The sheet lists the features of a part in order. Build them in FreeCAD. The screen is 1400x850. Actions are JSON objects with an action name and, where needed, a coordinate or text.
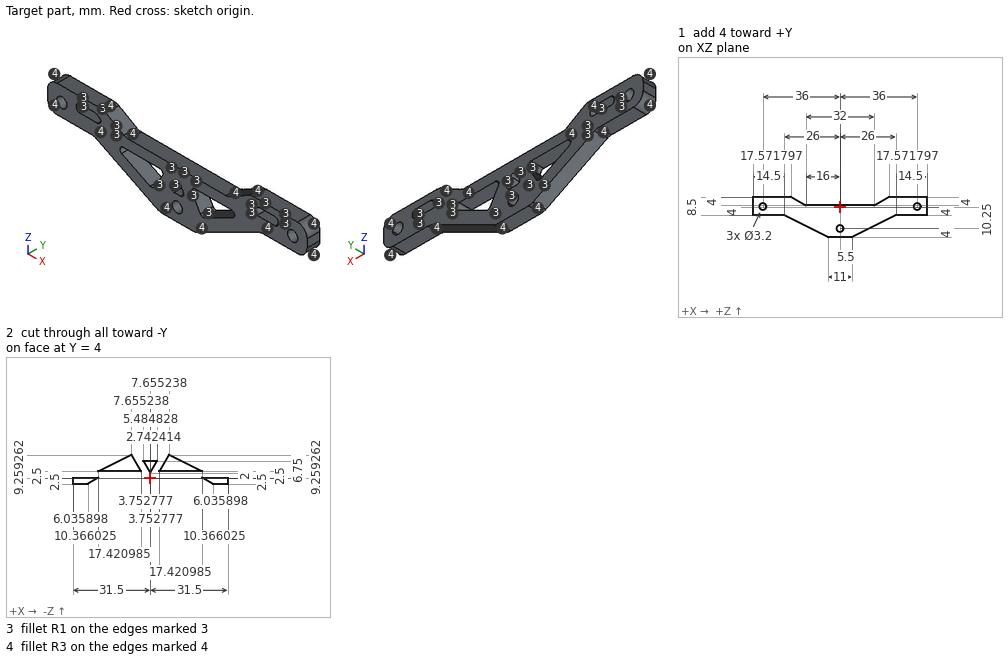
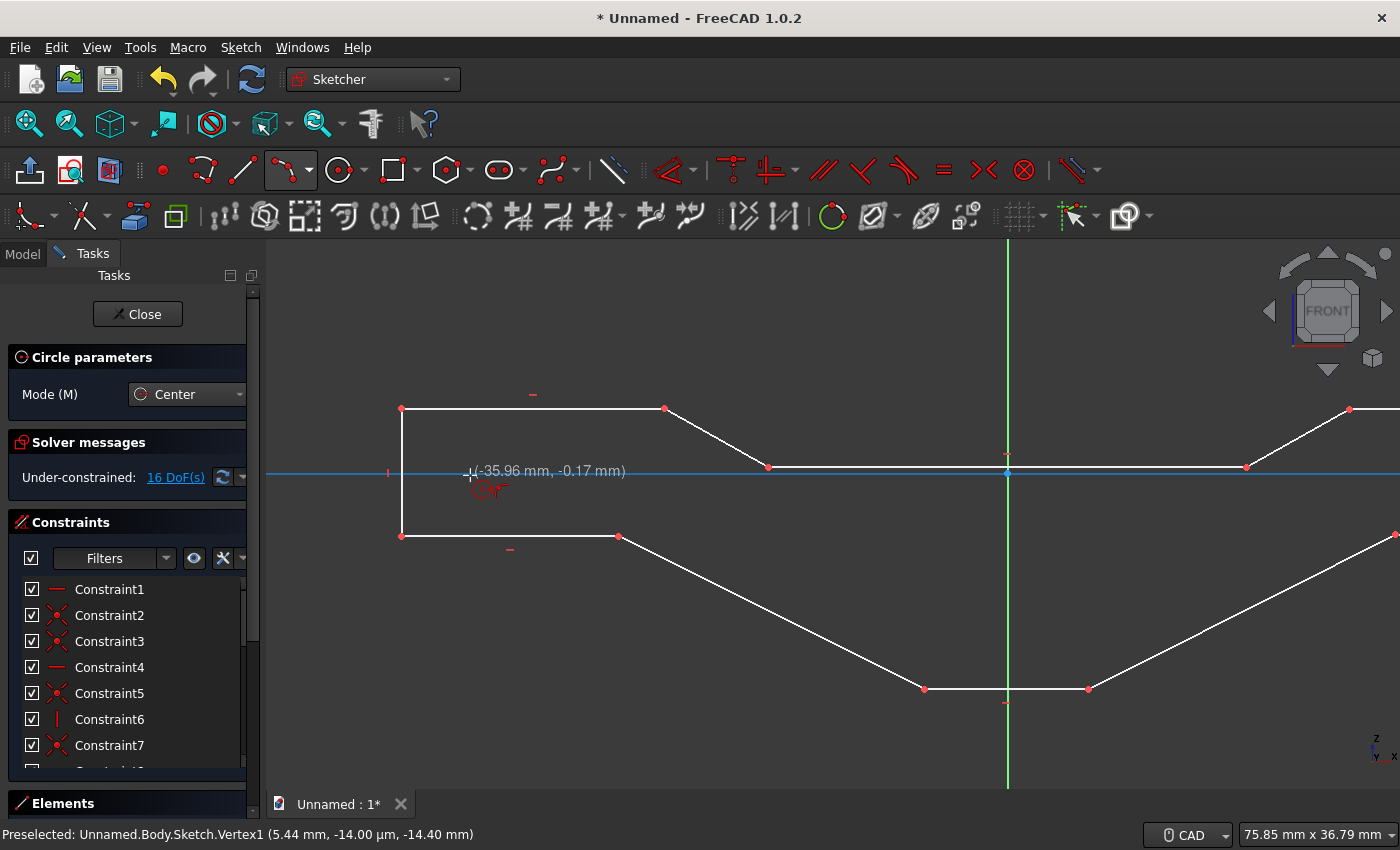
{"action": "left_click", "coordinate": [469, 474]}
{"action": "left_click", "coordinate": [486, 457]}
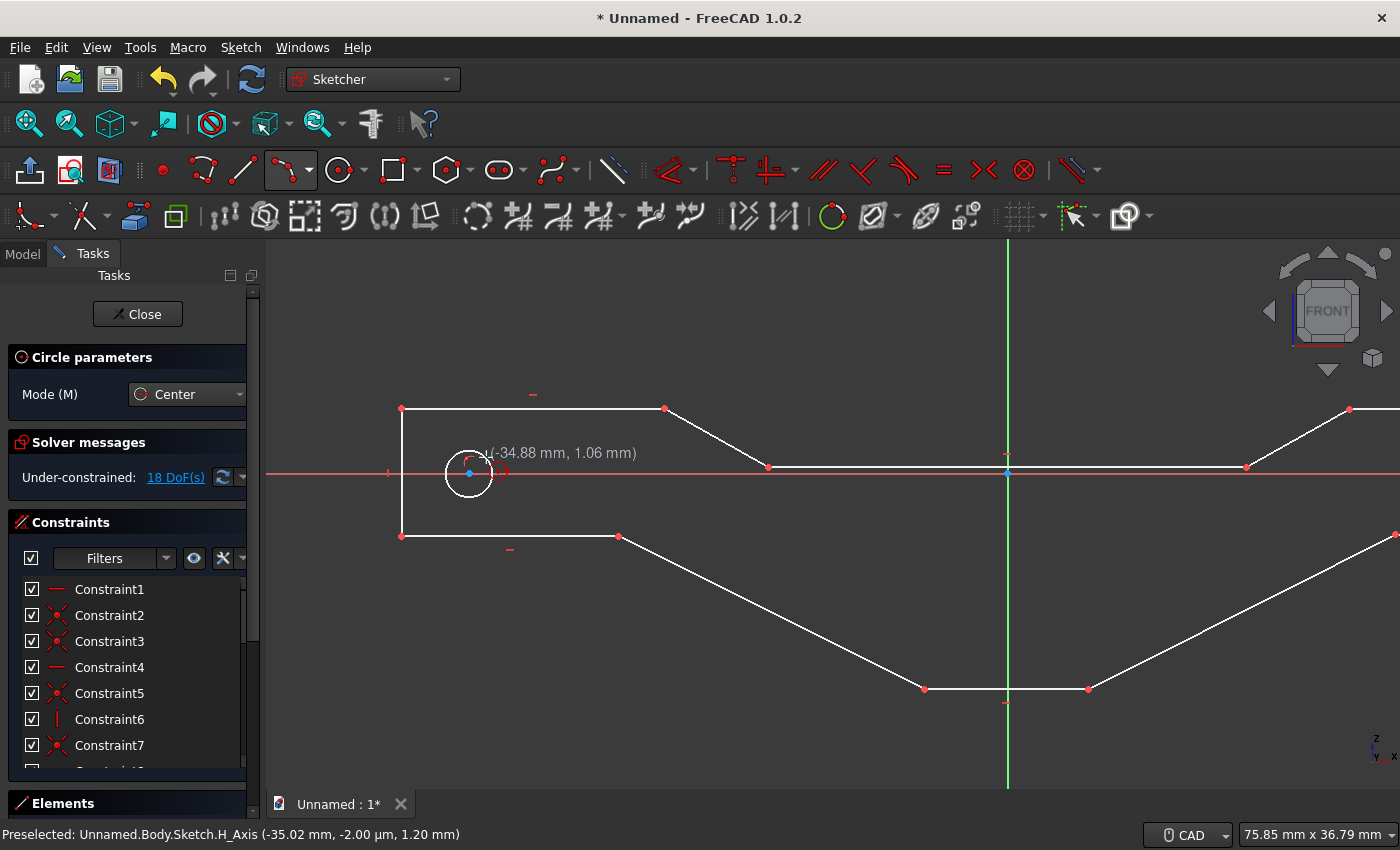
{"action": "scroll", "coordinate": [469, 474], "scroll_direction": "down", "scroll_amount": 3}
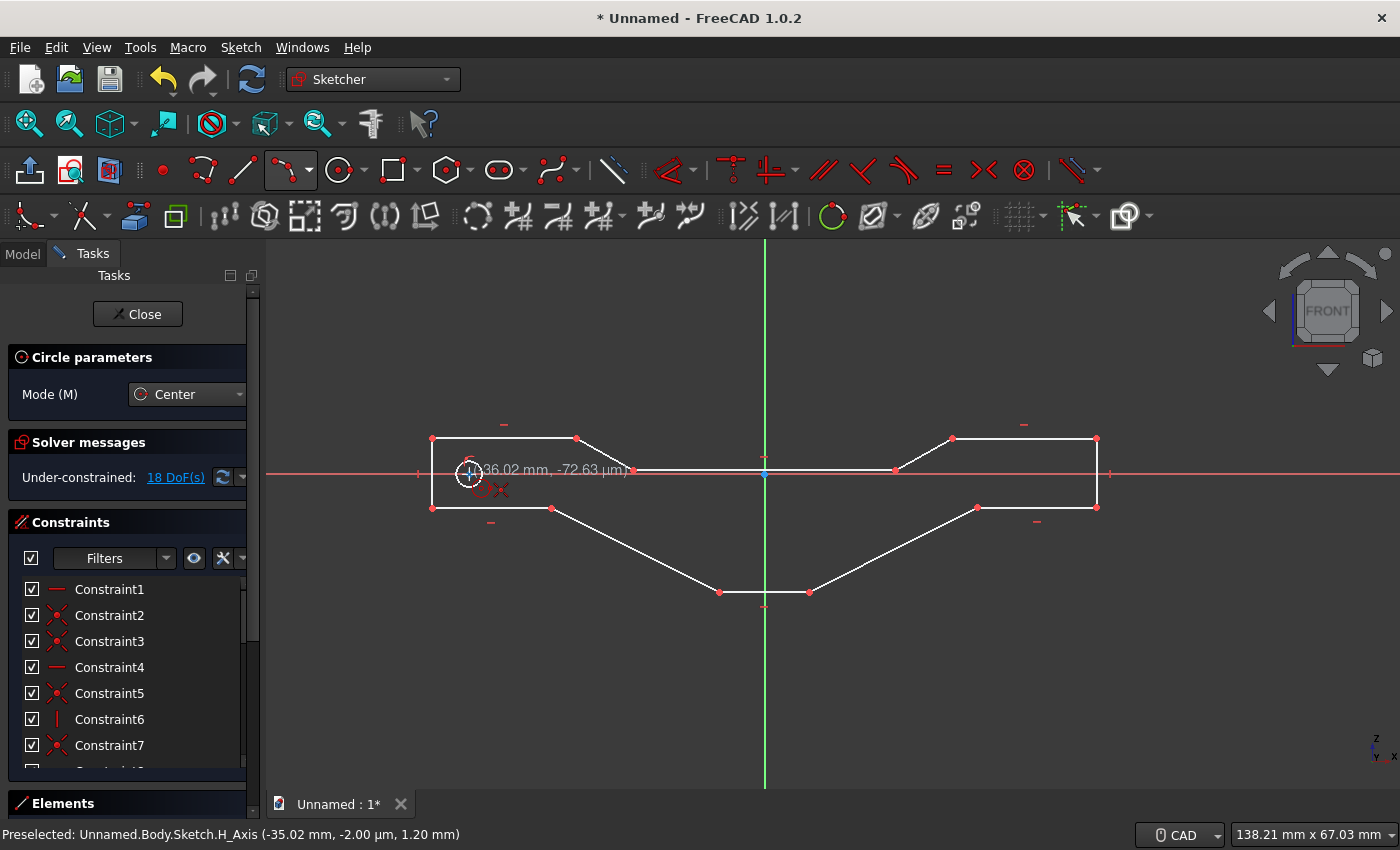
{"action": "scroll", "coordinate": [1060, 474], "scroll_direction": "up", "scroll_amount": 3}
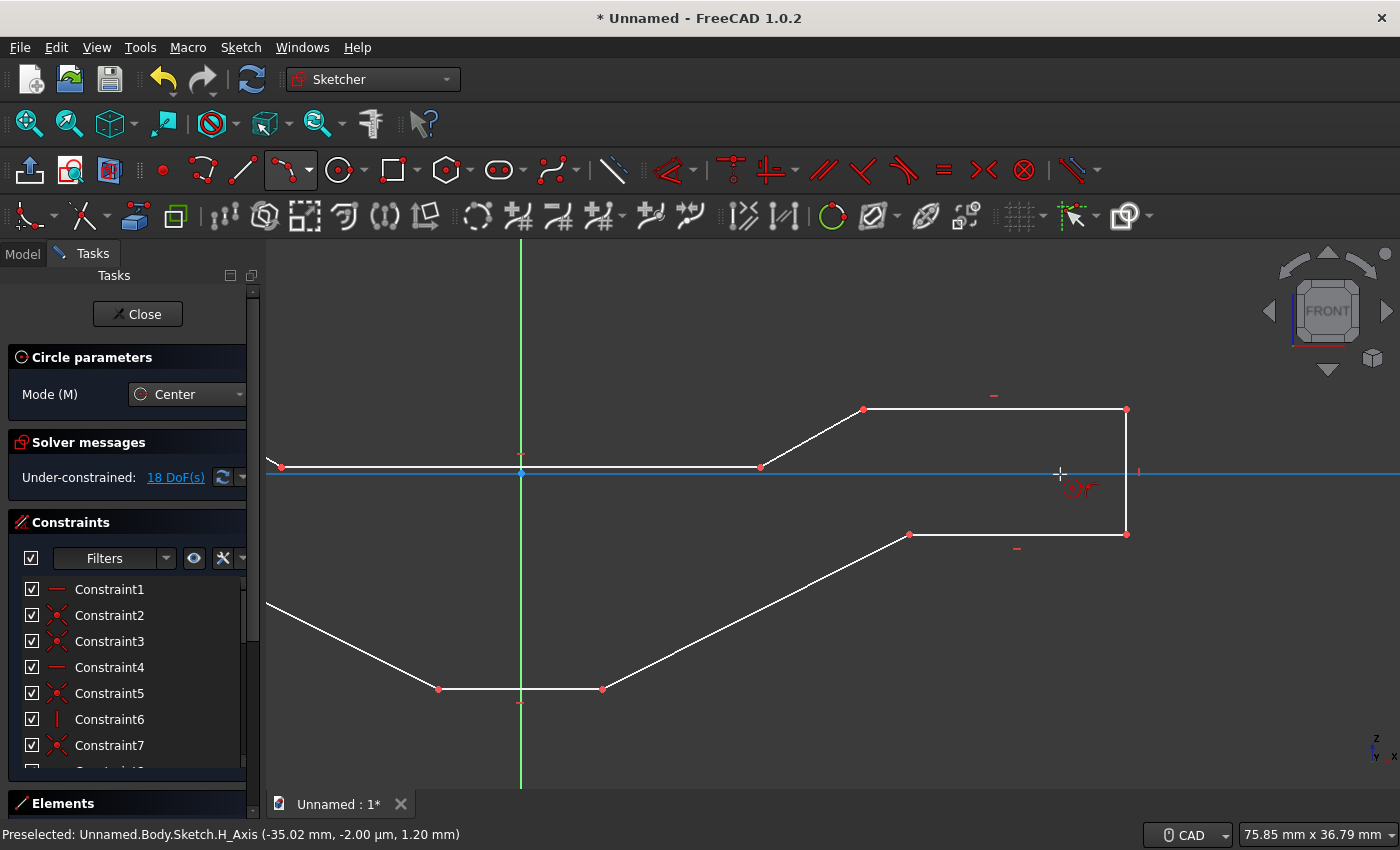
{"action": "left_click", "coordinate": [1059, 474]}
{"action": "left_click", "coordinate": [1076, 457]}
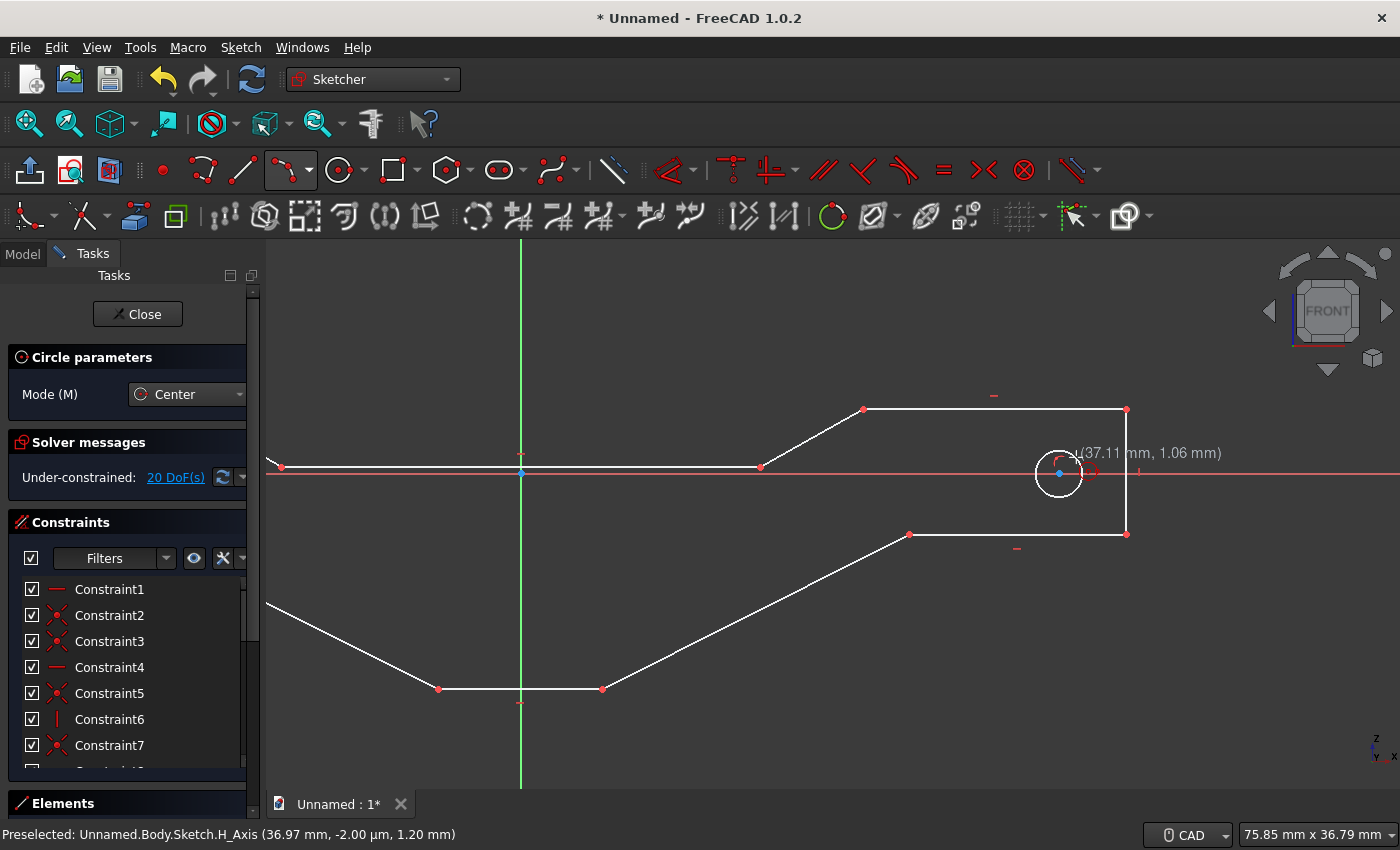
{"action": "left_click", "coordinate": [521, 627]}
{"action": "left_click", "coordinate": [538, 610]}
{"action": "key", "text": "Escape"}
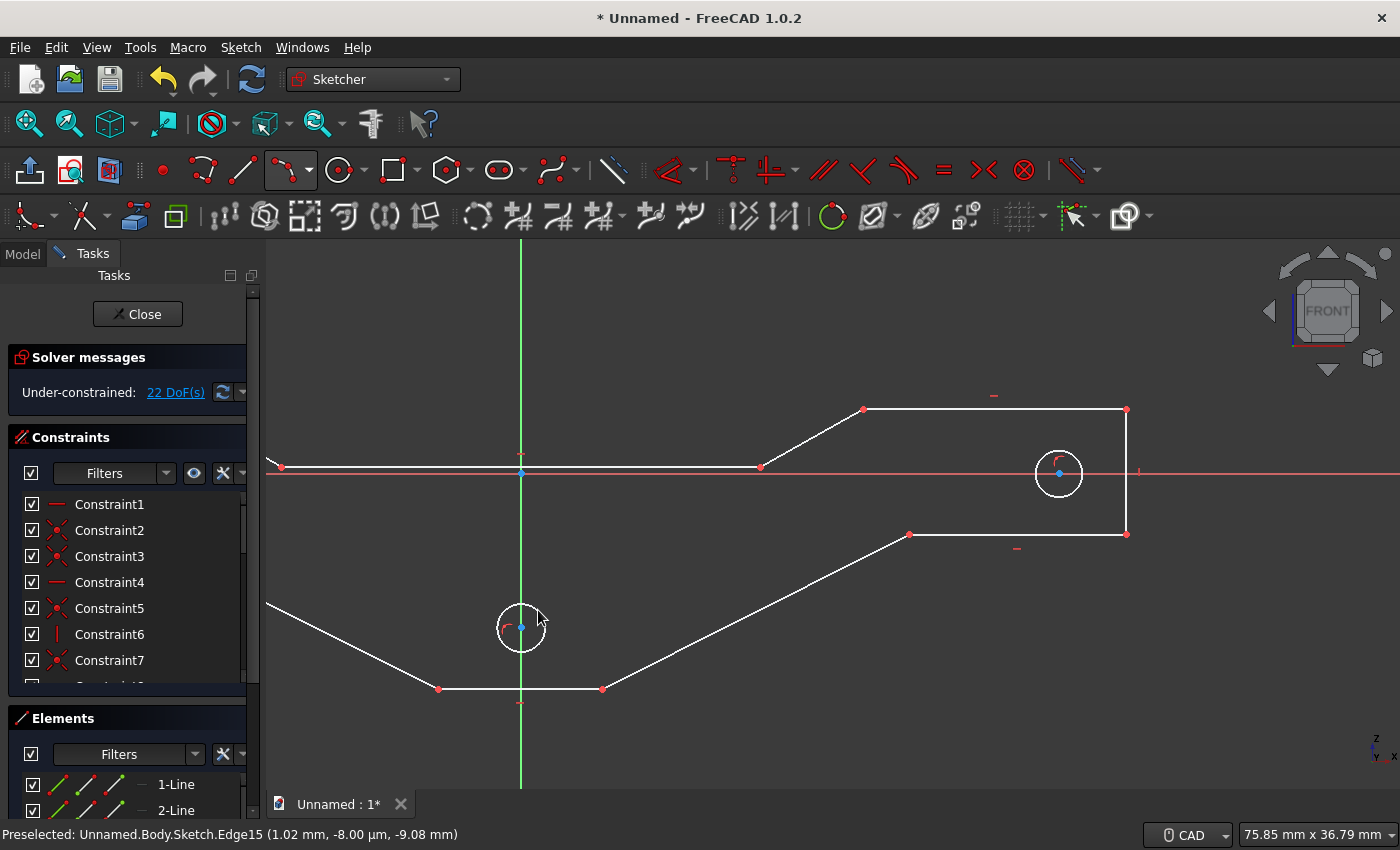
{"action": "scroll", "coordinate": [1060, 474], "scroll_direction": "down", "scroll_amount": 3}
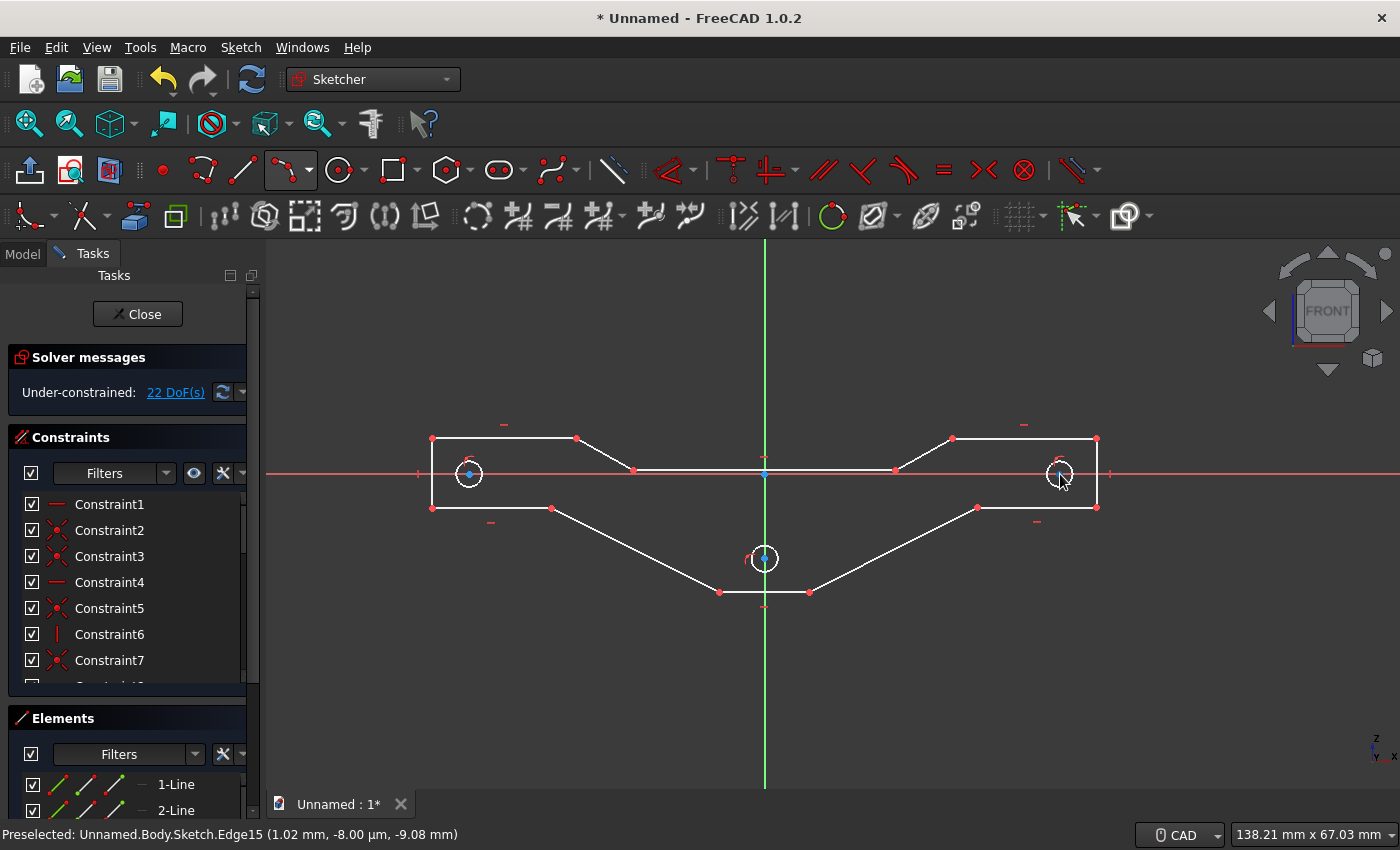
{"action": "scroll", "coordinate": [478, 465], "scroll_direction": "up", "scroll_amount": 3}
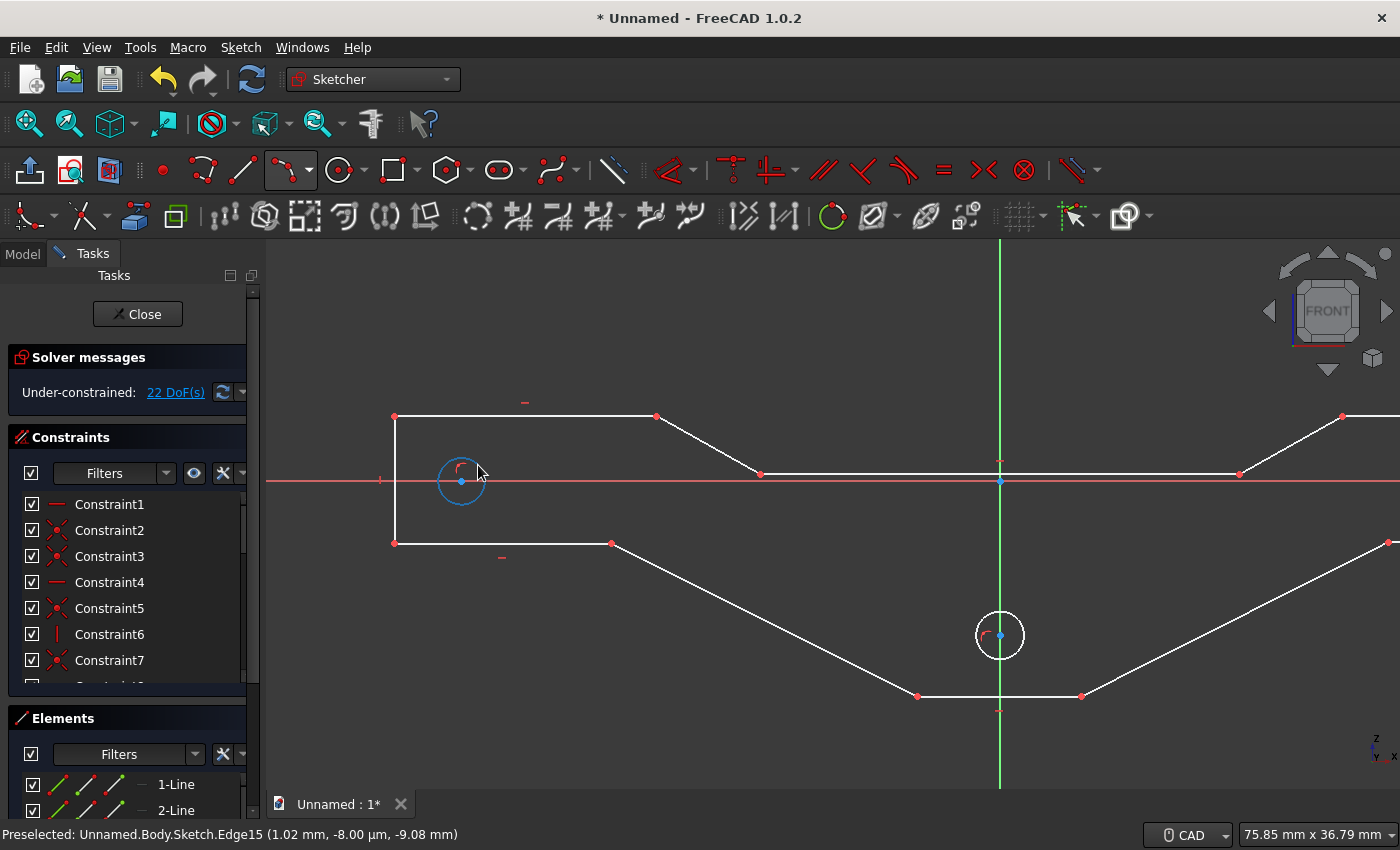
{"action": "left_click", "coordinate": [478, 465]}